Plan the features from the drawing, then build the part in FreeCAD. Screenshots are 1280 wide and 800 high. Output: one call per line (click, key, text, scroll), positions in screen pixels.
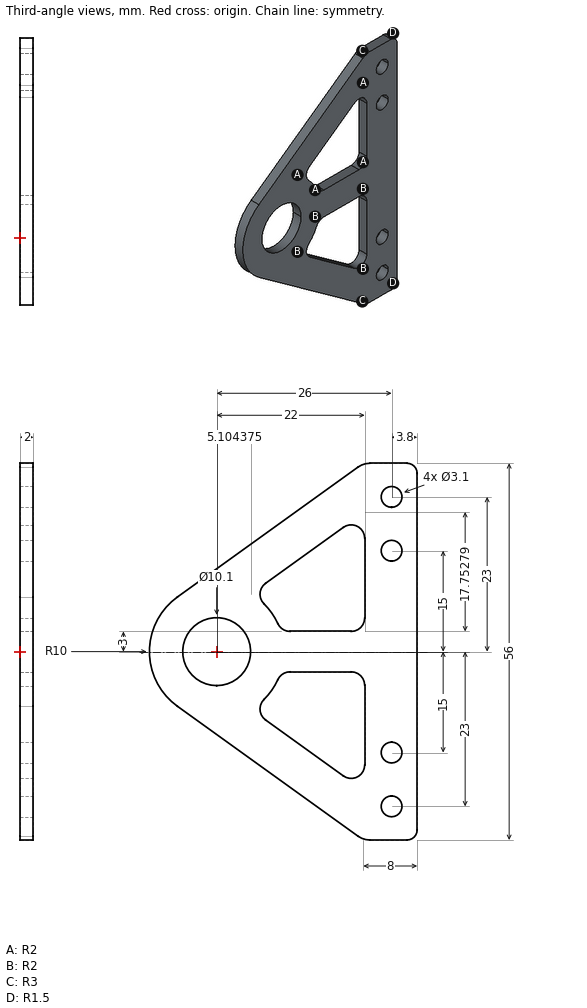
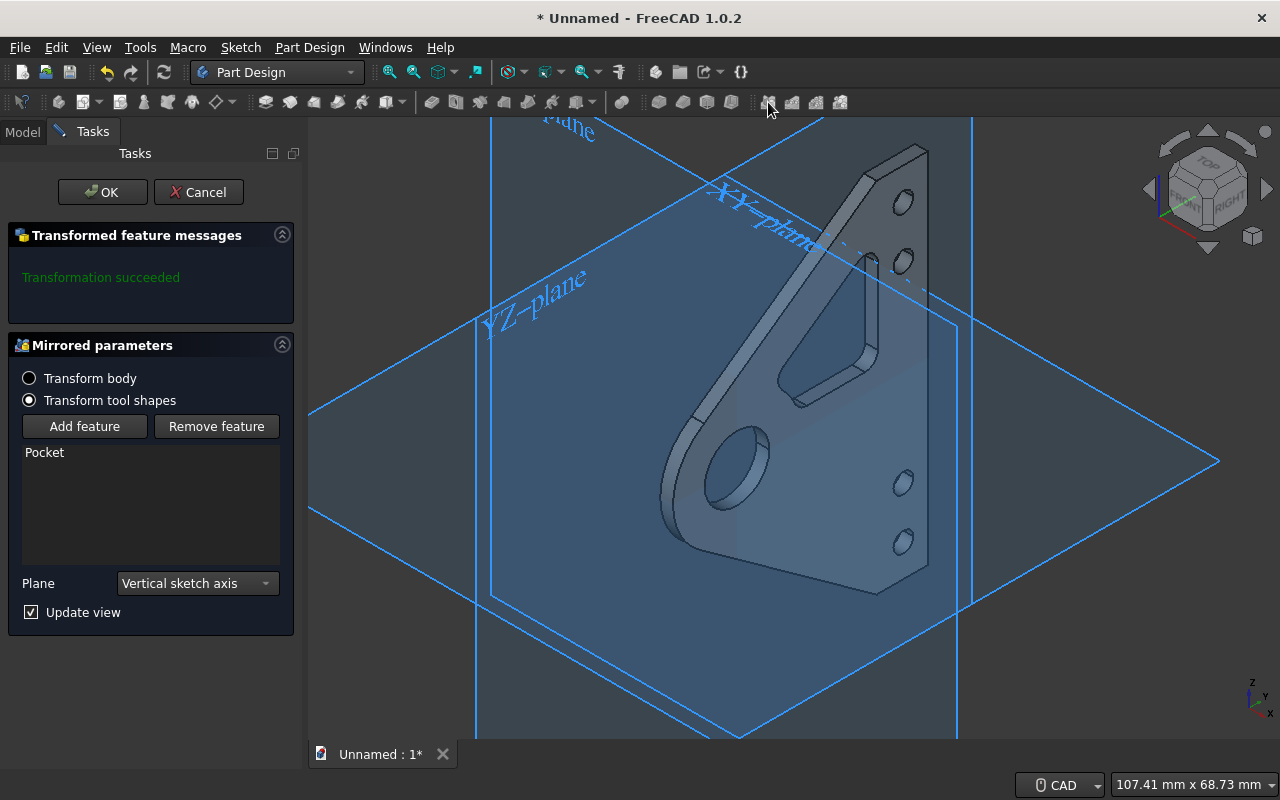
click(198, 584)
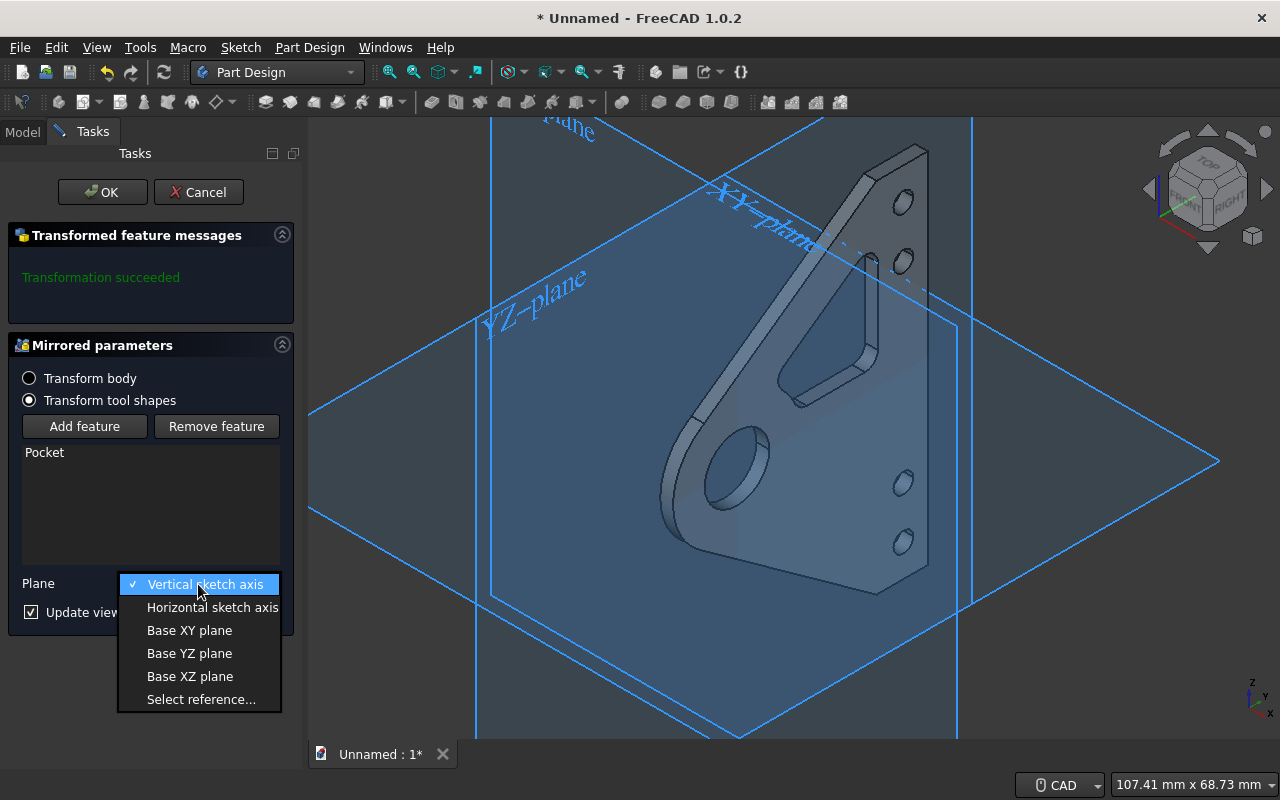
click(198, 630)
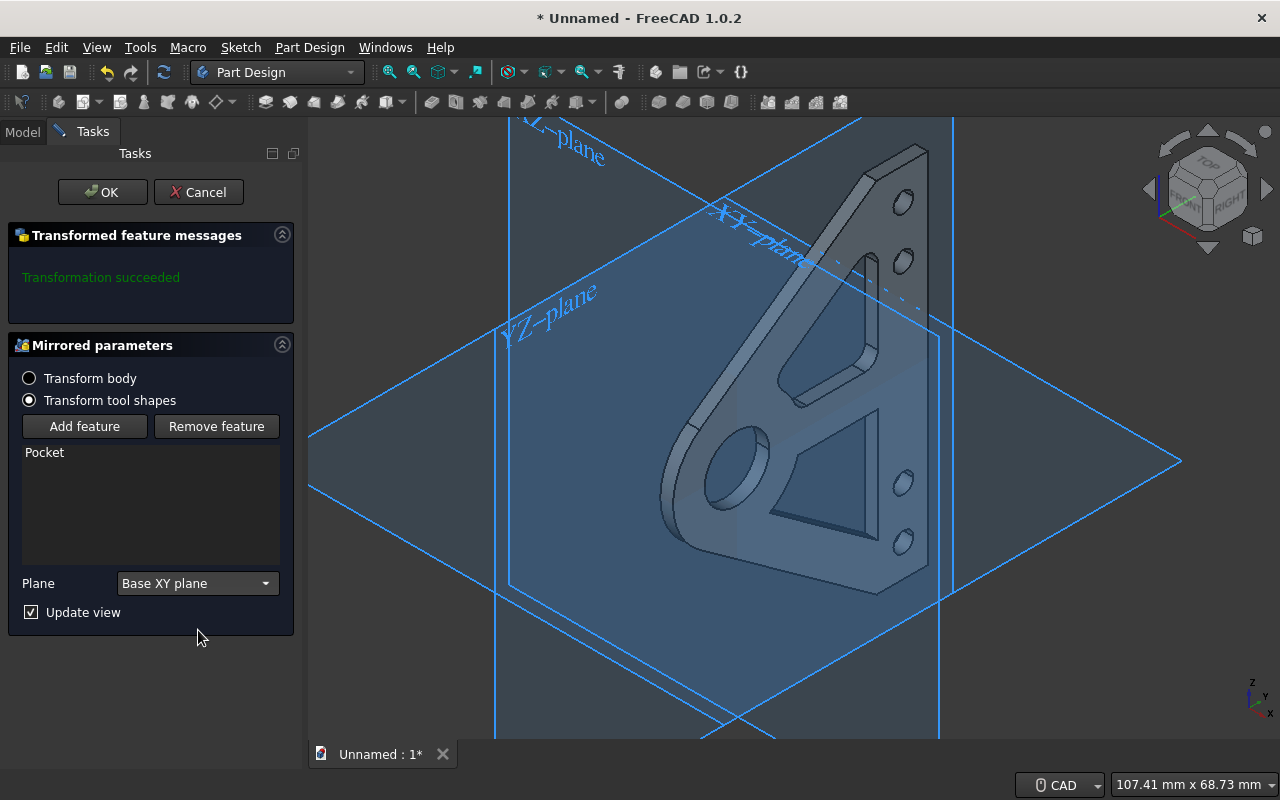
click(103, 192)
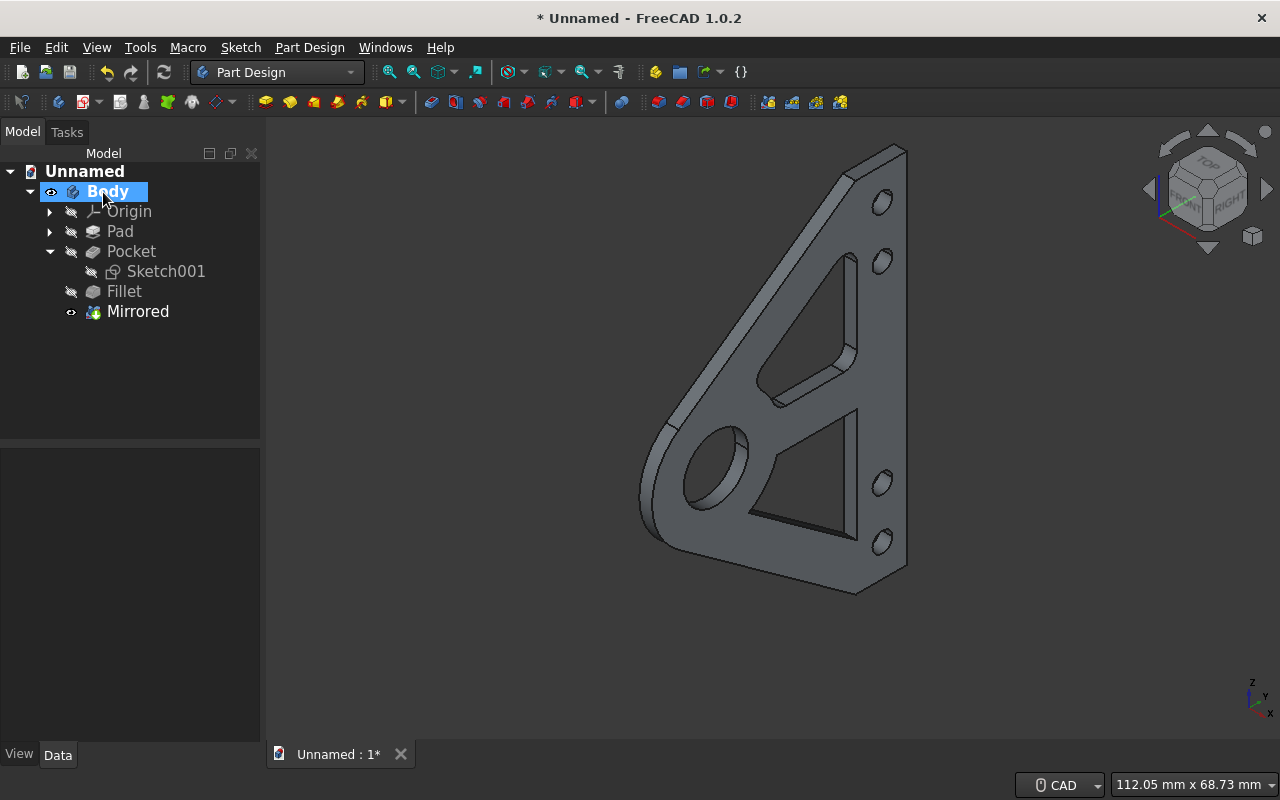
scroll(850, 536, up, 4)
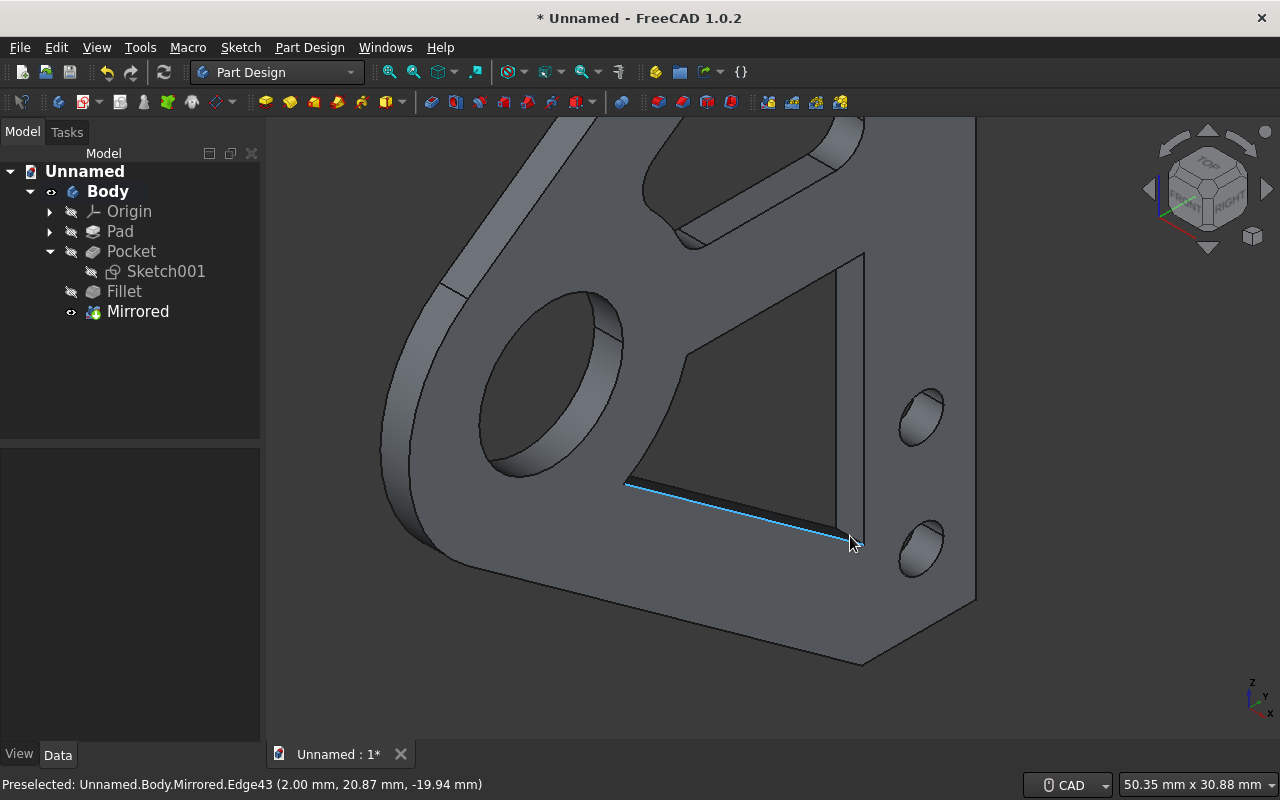
click(390, 72)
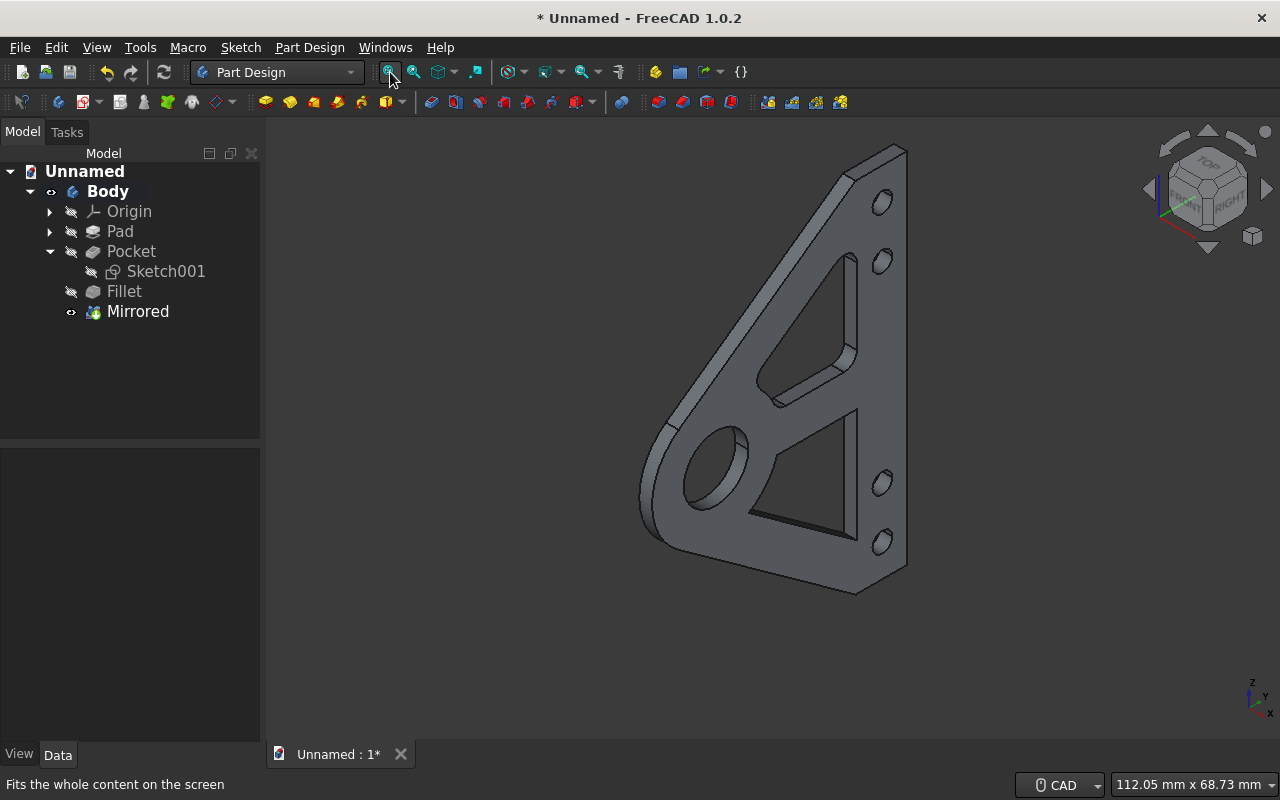
key(2)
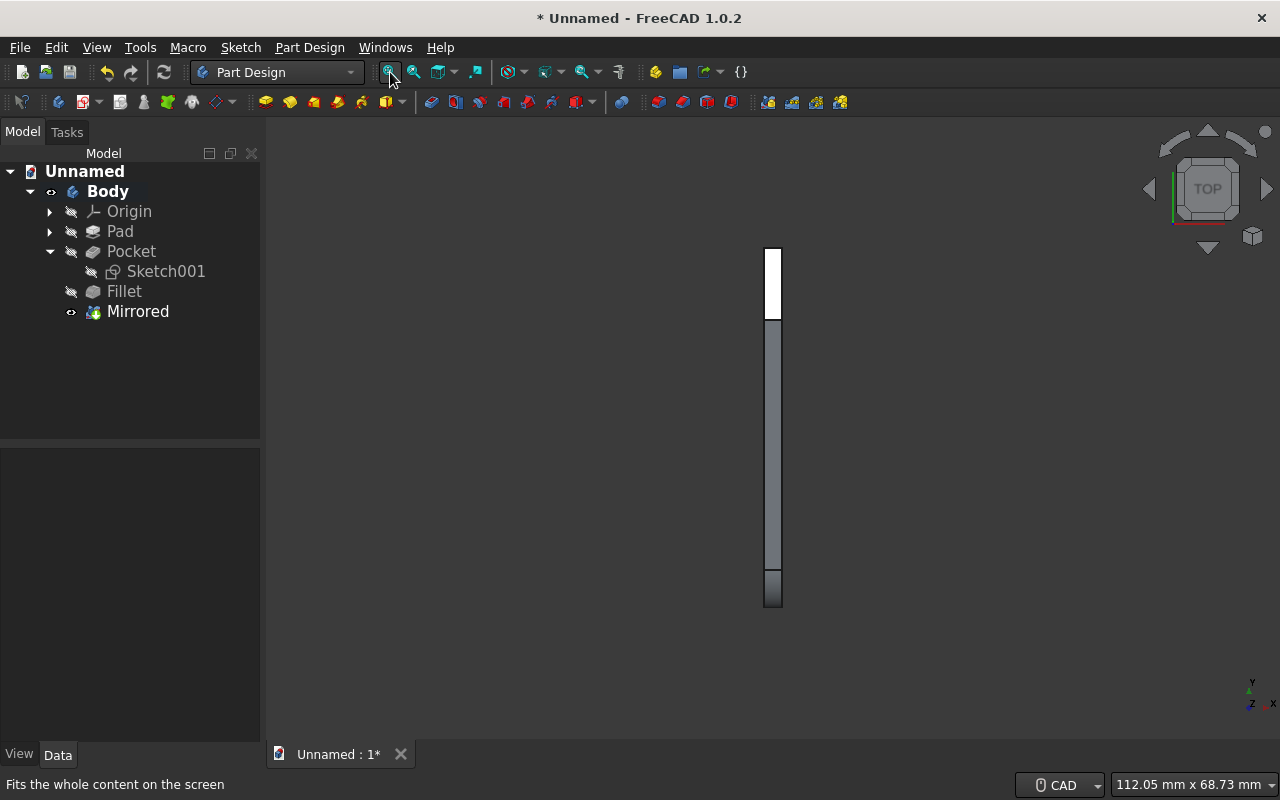
scroll(773, 317, up, 4)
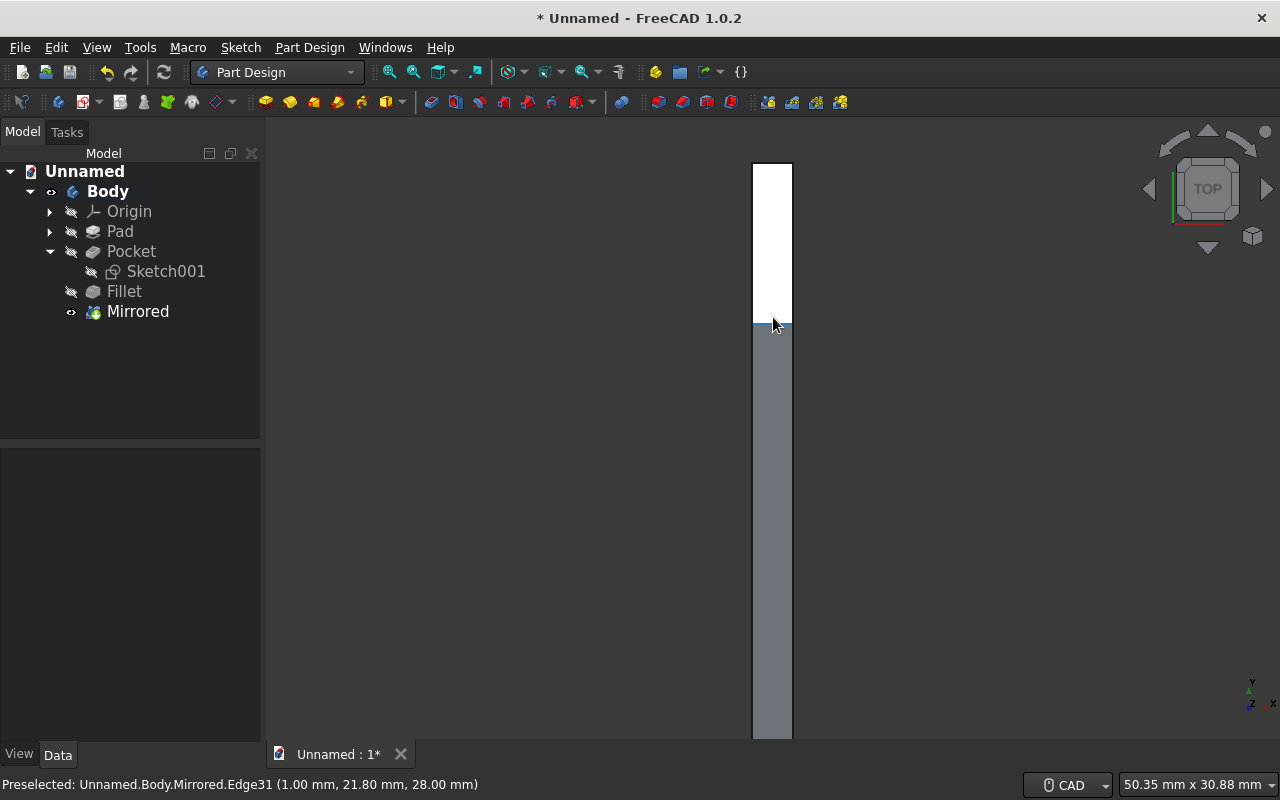
click(390, 72)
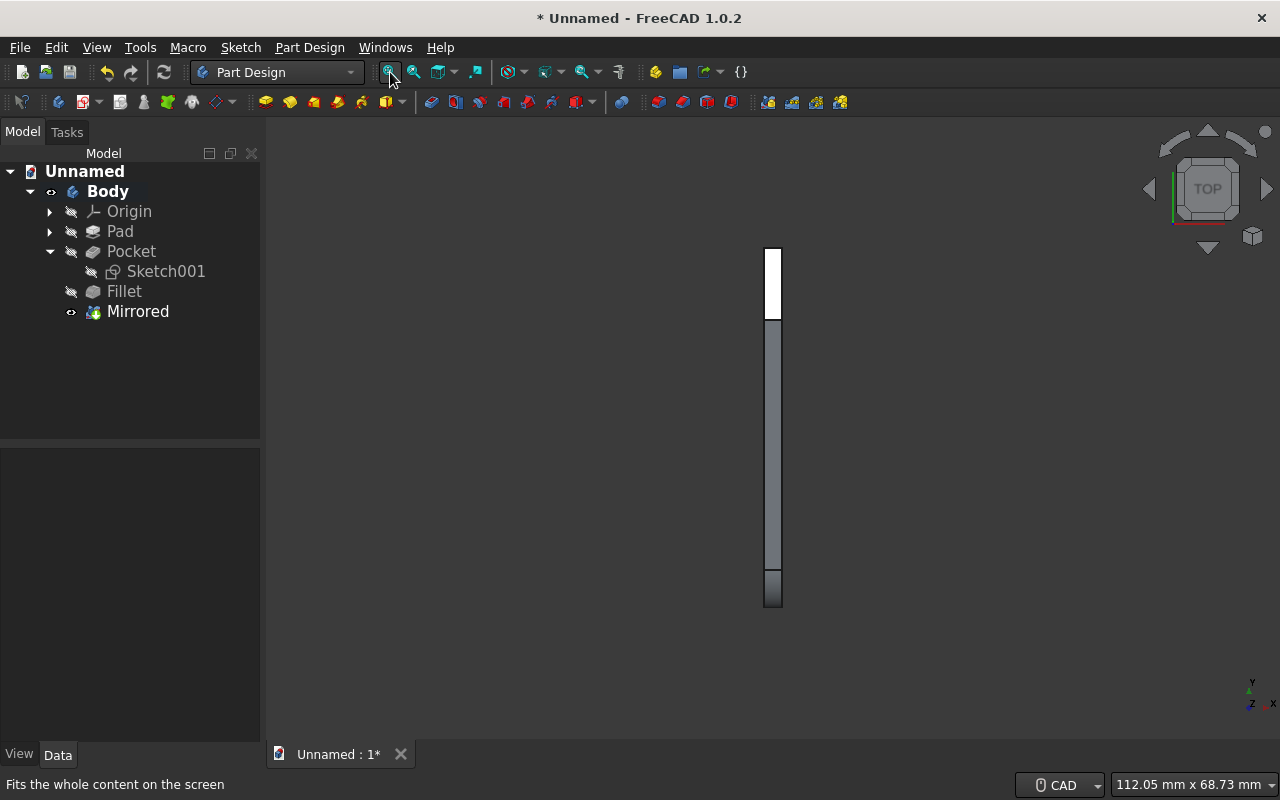
key(0)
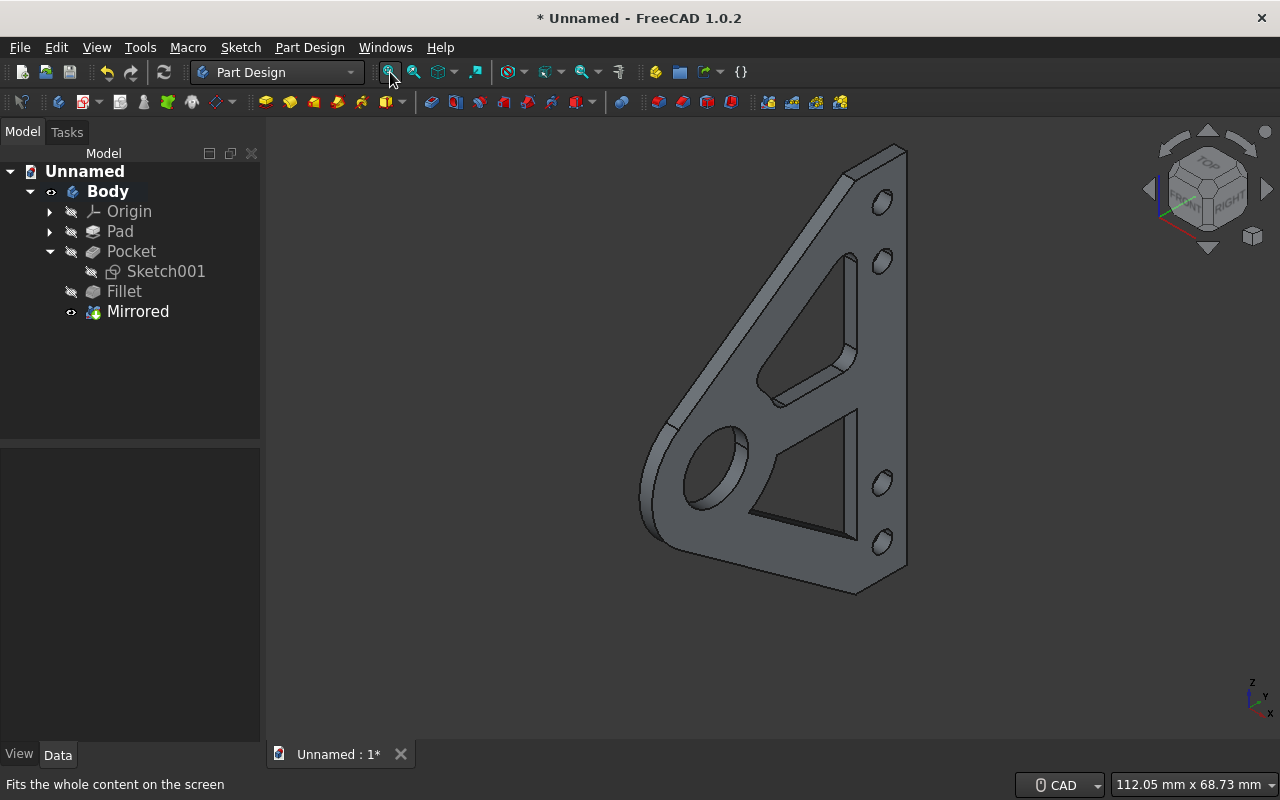
scroll(850, 536, up, 4)